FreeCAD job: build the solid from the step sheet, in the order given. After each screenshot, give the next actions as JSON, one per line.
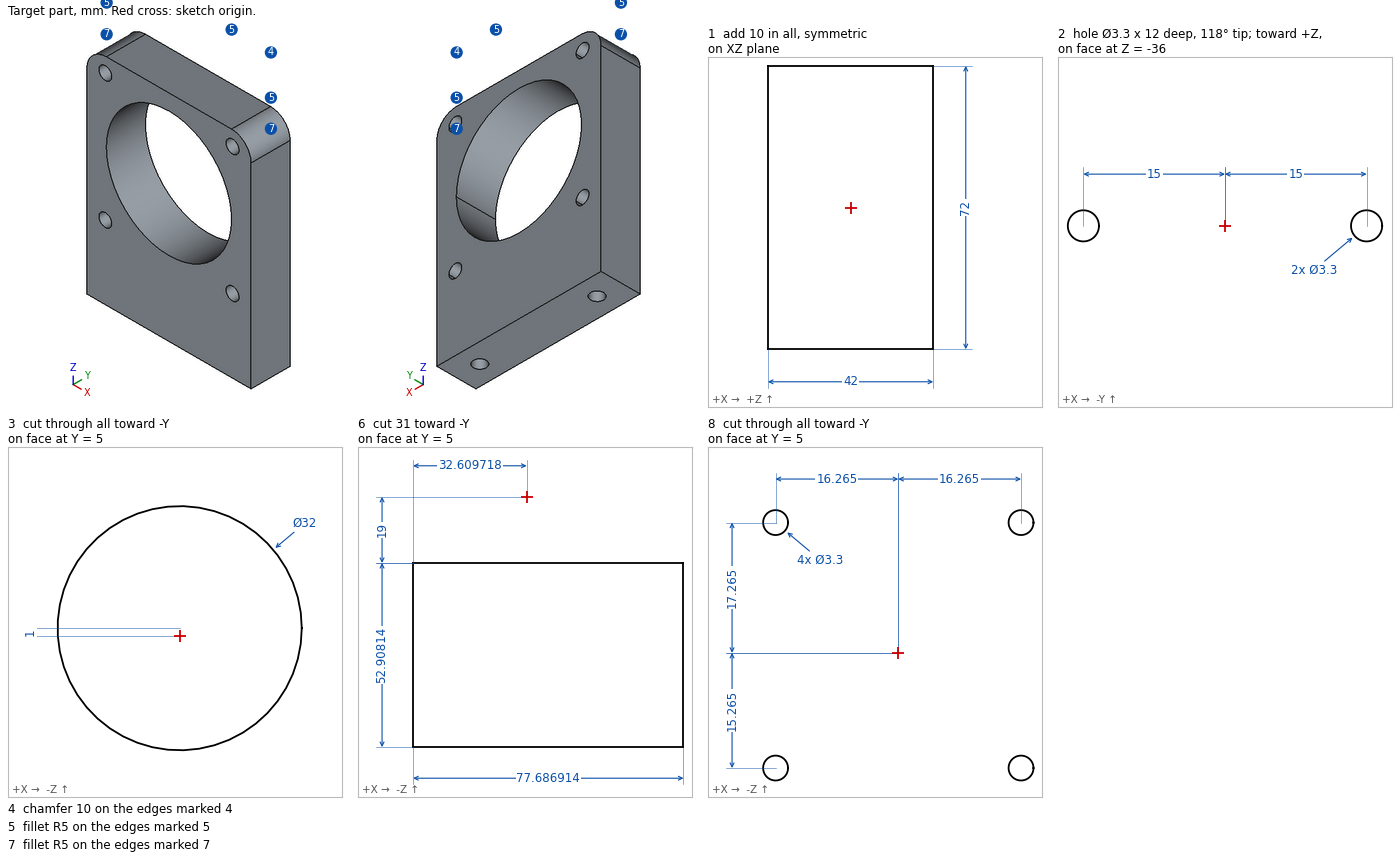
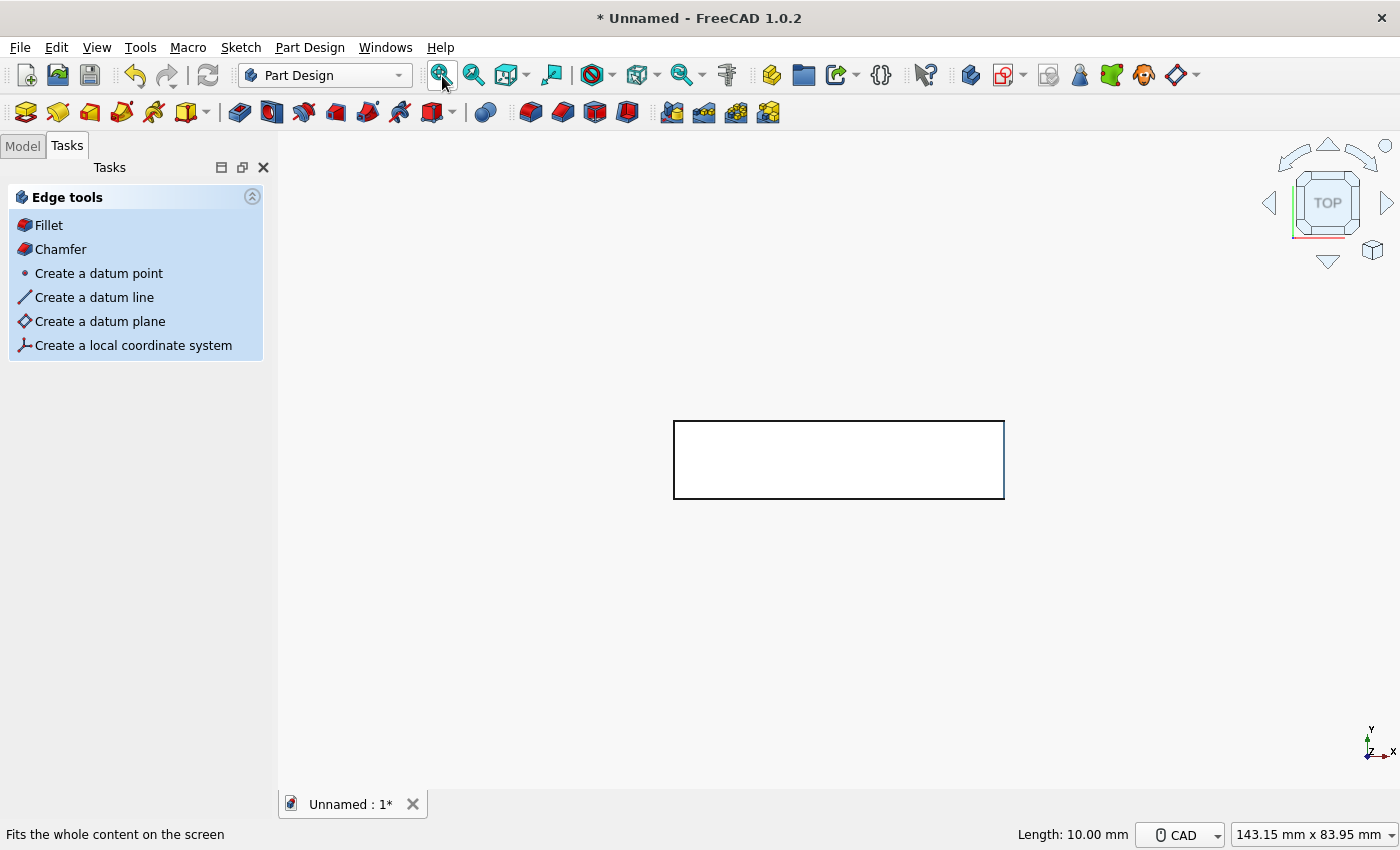
{"action": "left_click", "coordinate": [674, 459], "text": "ctrl"}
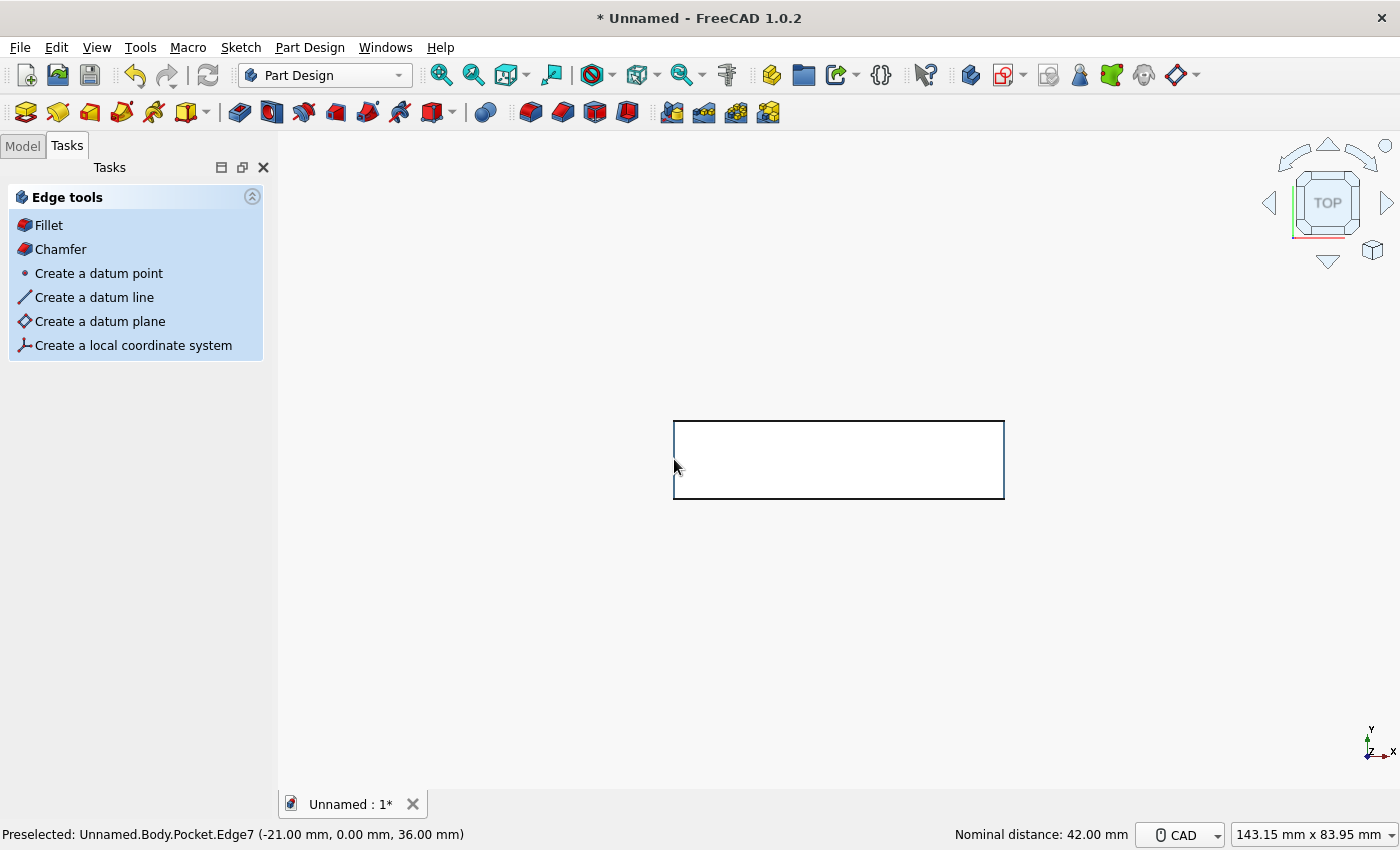
{"action": "left_click", "coordinate": [564, 112]}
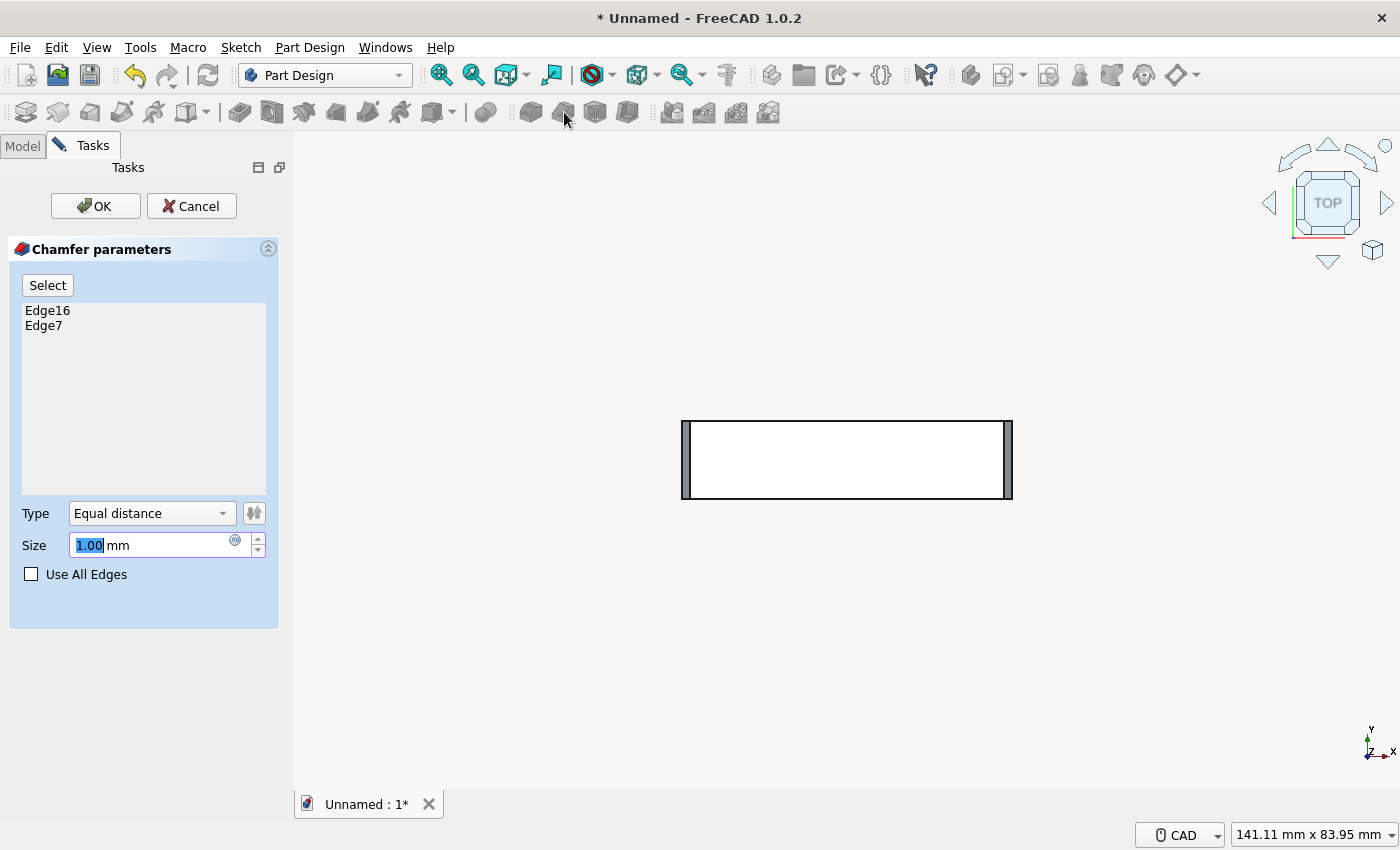
{"action": "type", "text": "10"}
{"action": "key", "text": "Tab"}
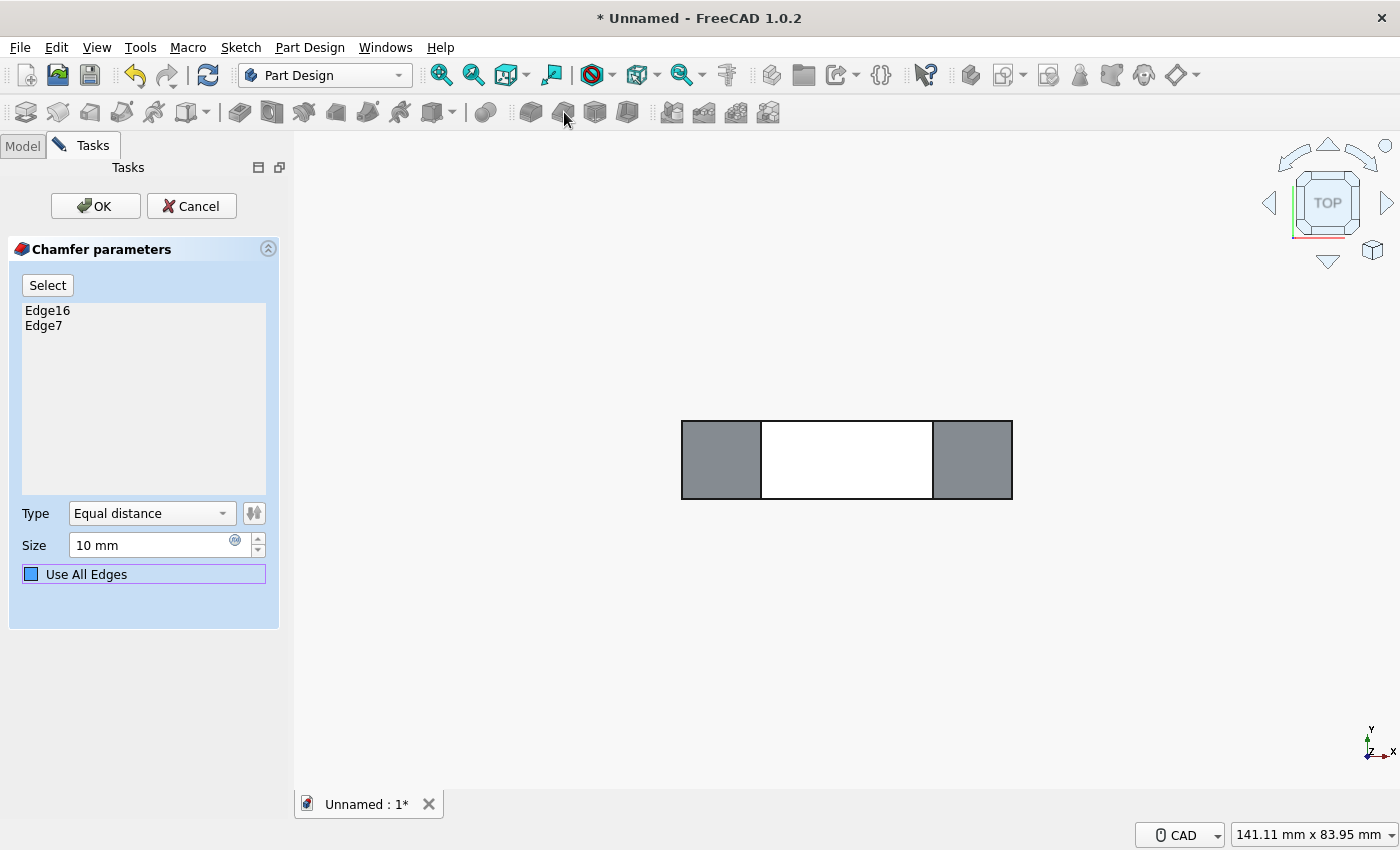
{"action": "left_click", "coordinate": [96, 206]}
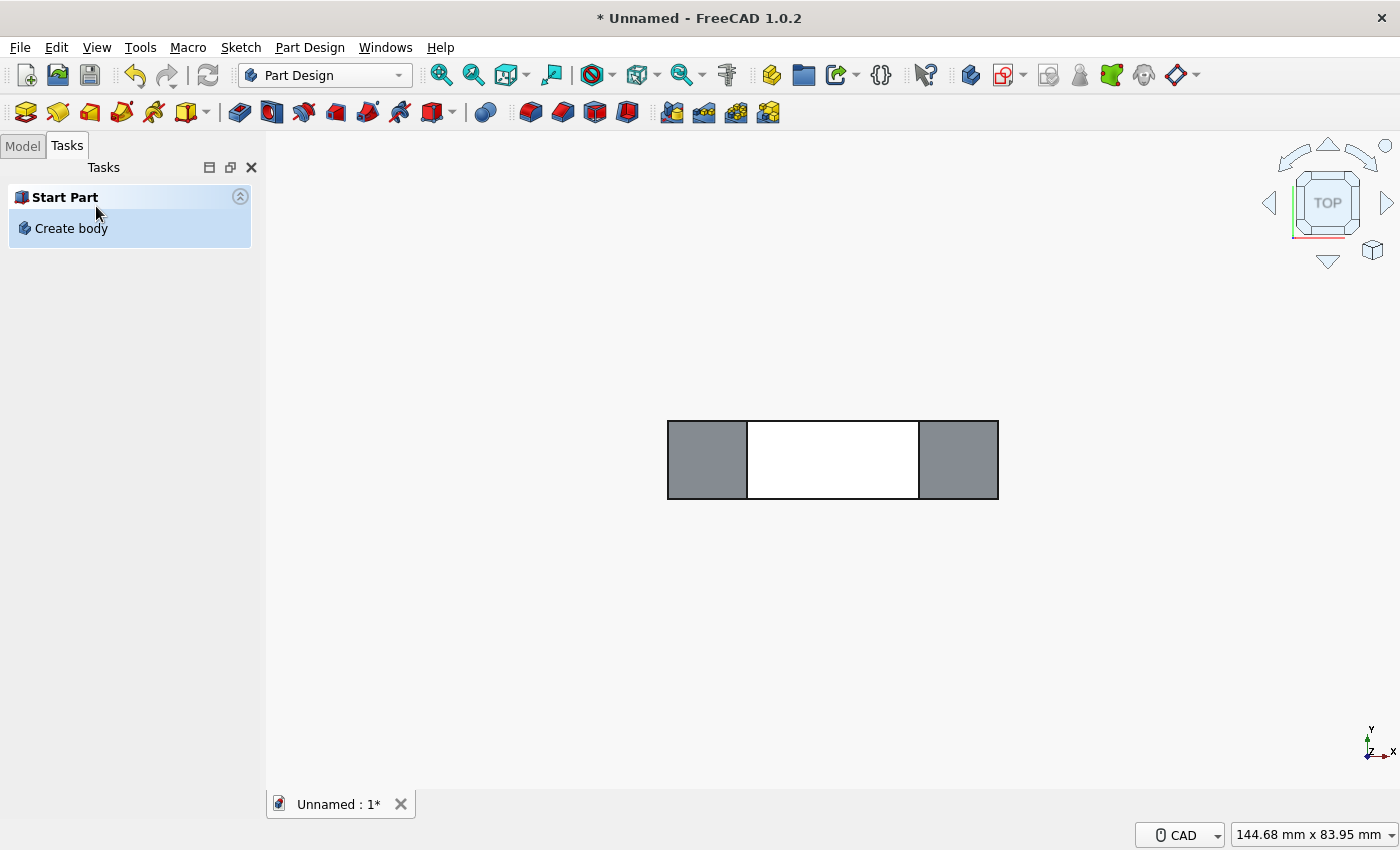
{"action": "left_click", "coordinate": [442, 76]}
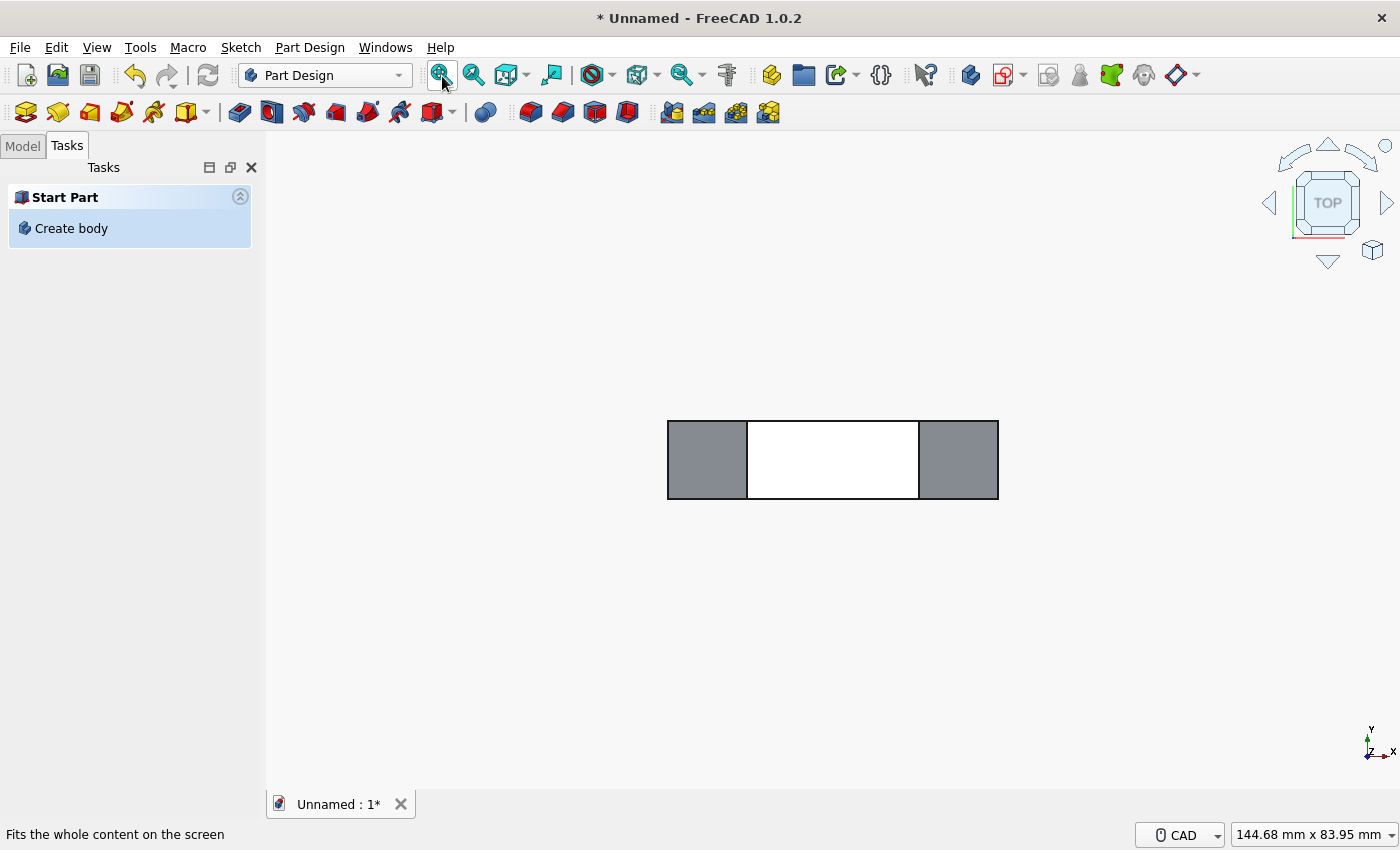
{"action": "left_click", "coordinate": [919, 459]}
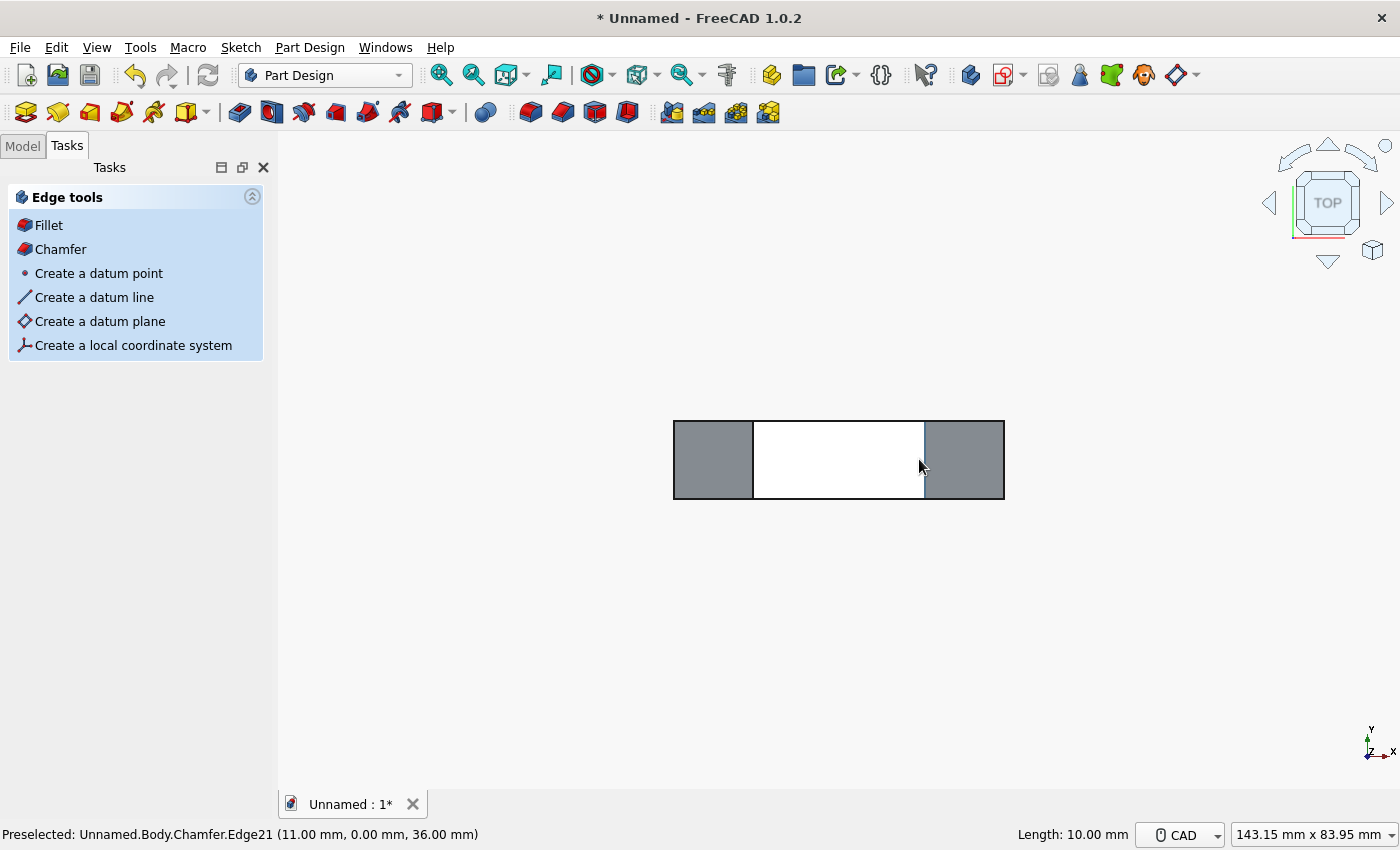
{"action": "left_click", "coordinate": [753, 459], "text": "ctrl"}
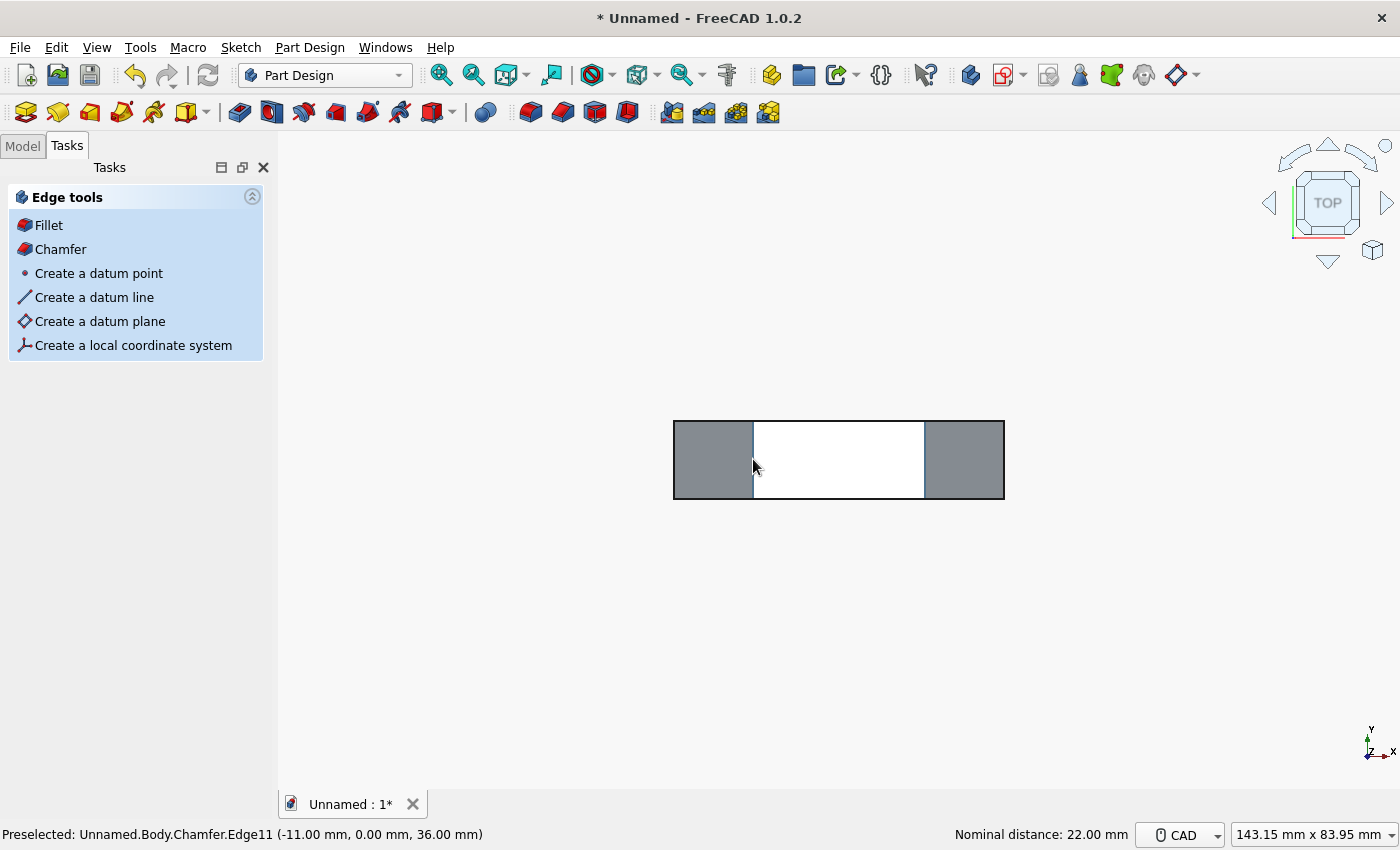
{"action": "key", "text": "0"}